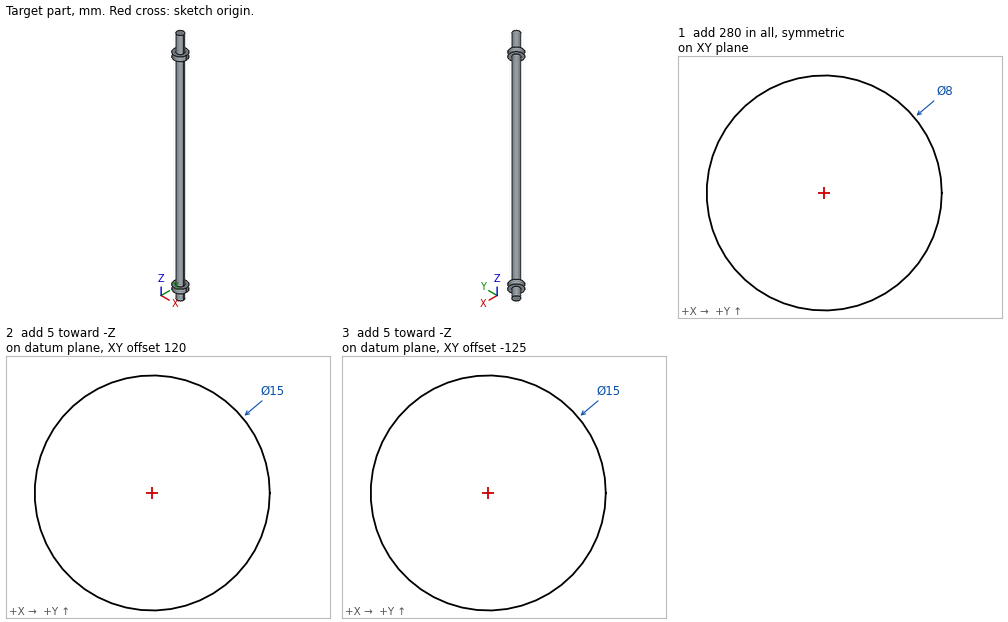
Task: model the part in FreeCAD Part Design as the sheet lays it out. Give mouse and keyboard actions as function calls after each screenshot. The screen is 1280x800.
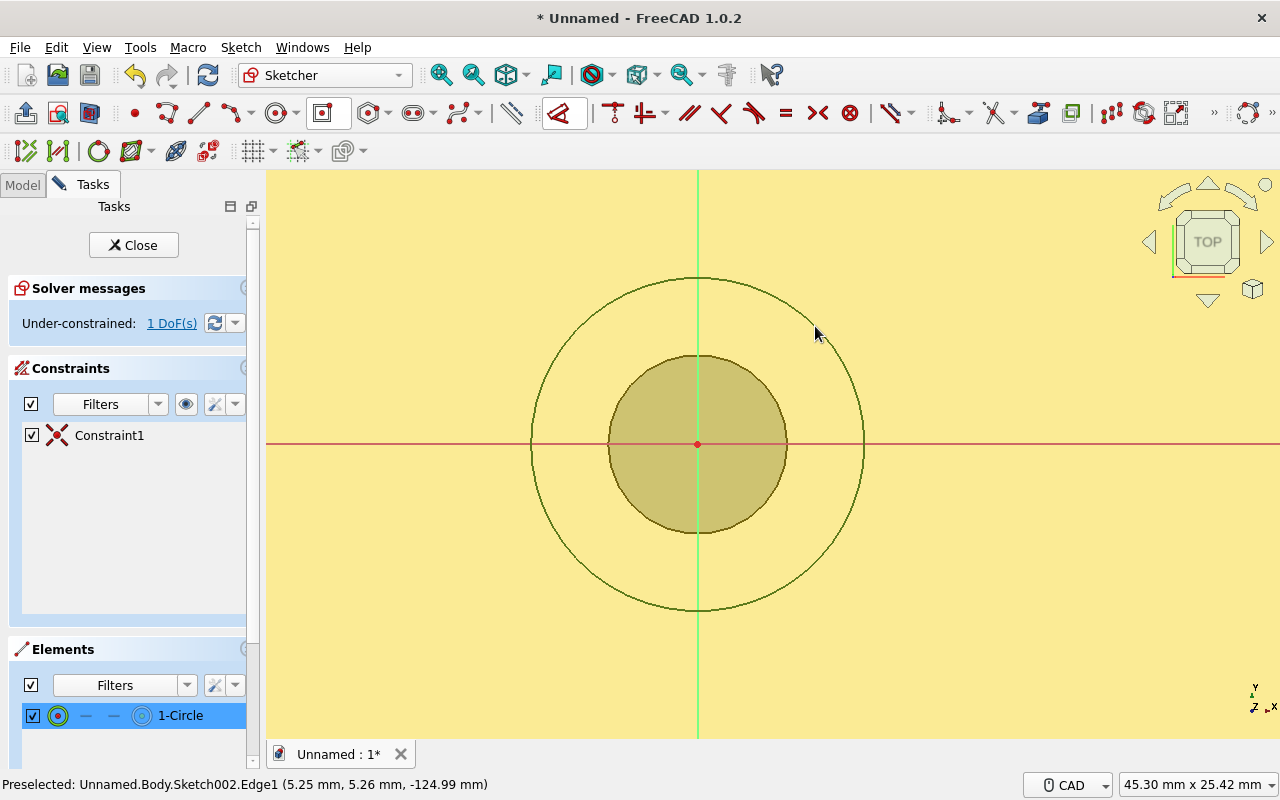
key(k)
key(o)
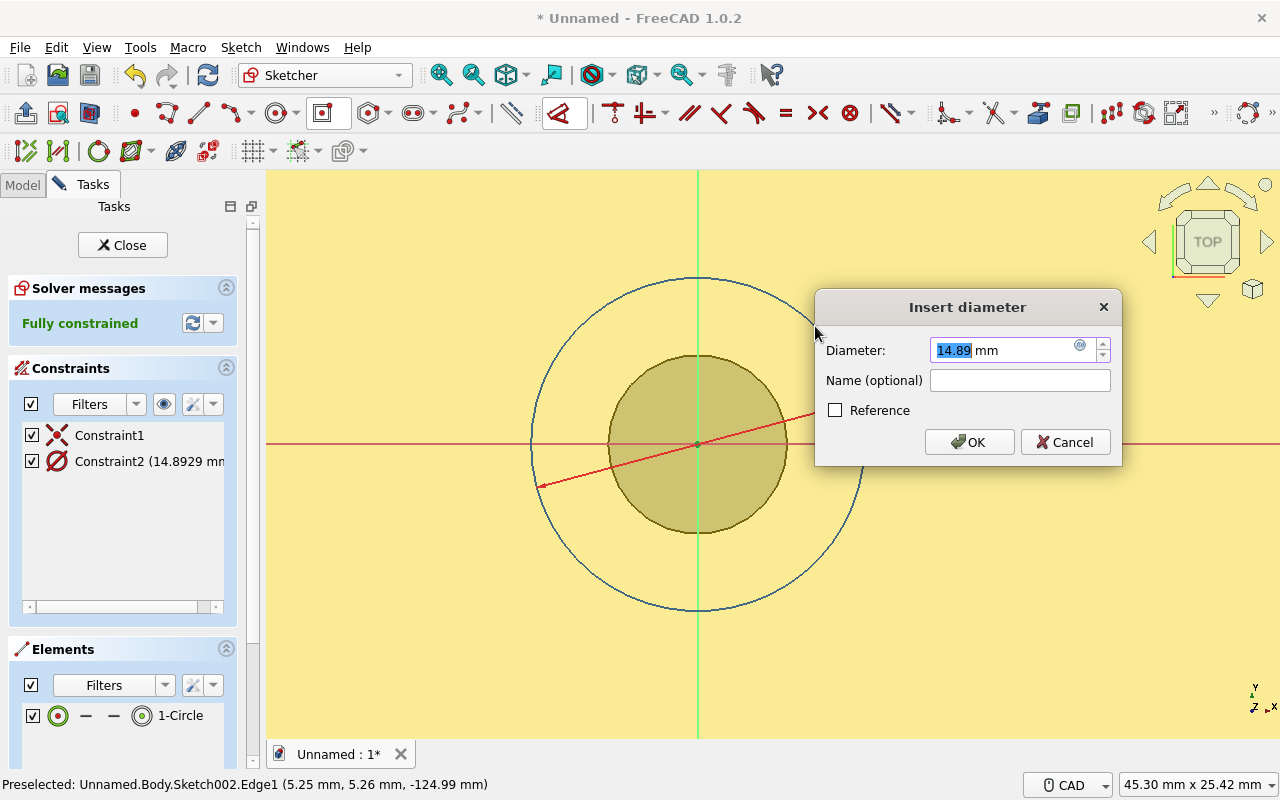
text(15)
key(Return)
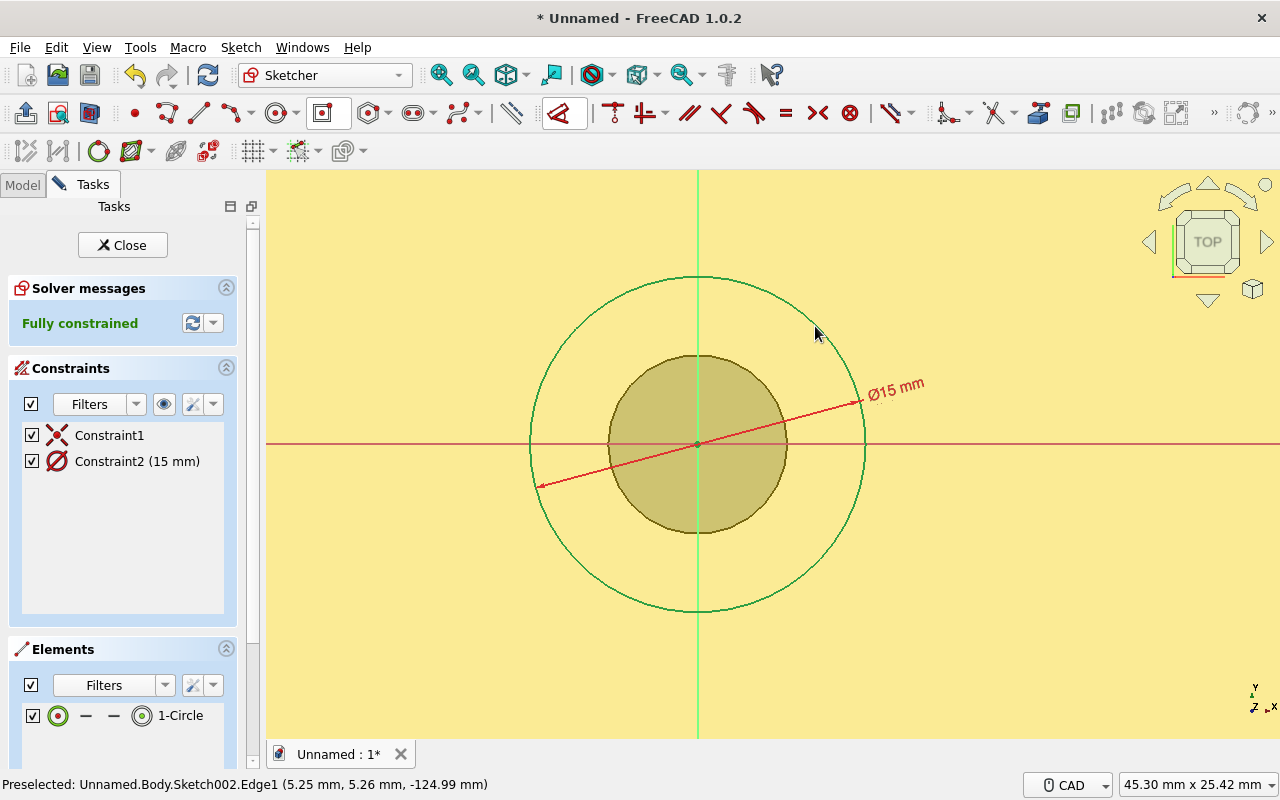
click(123, 245)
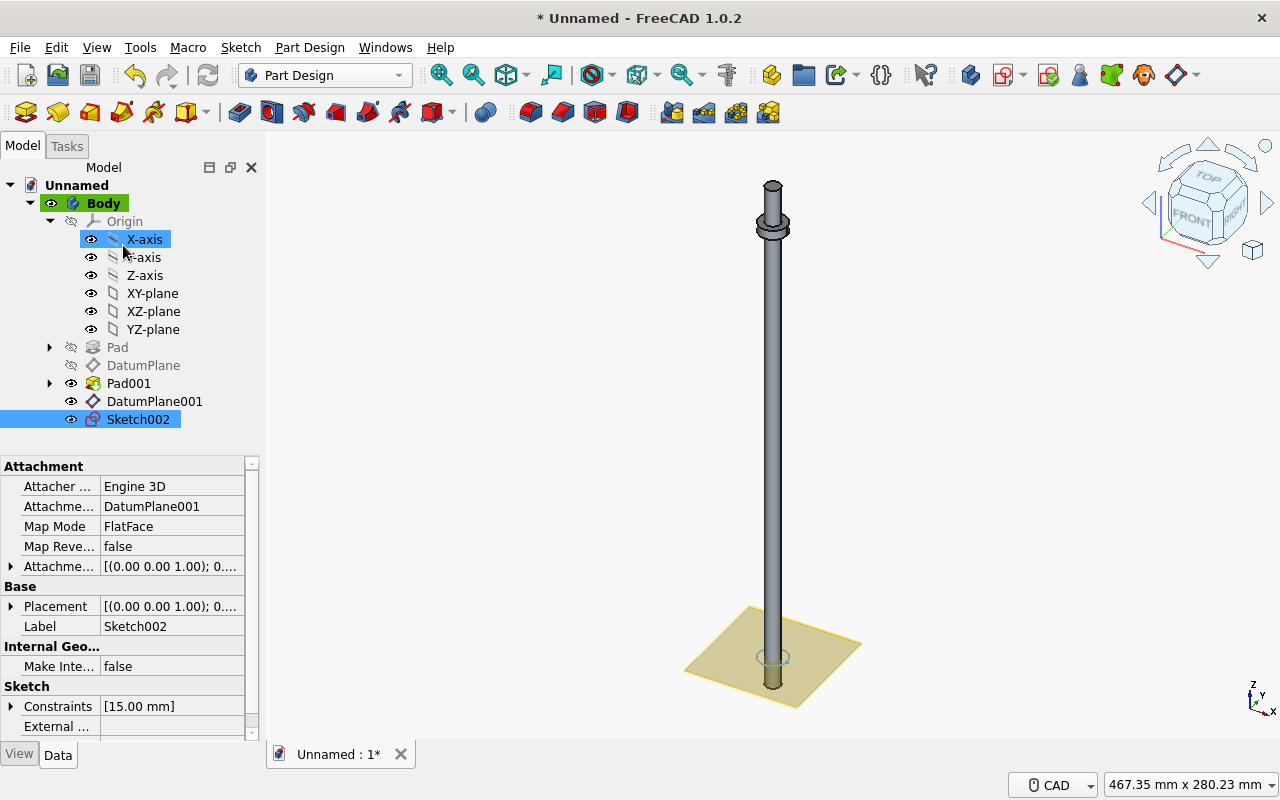
click(26, 112)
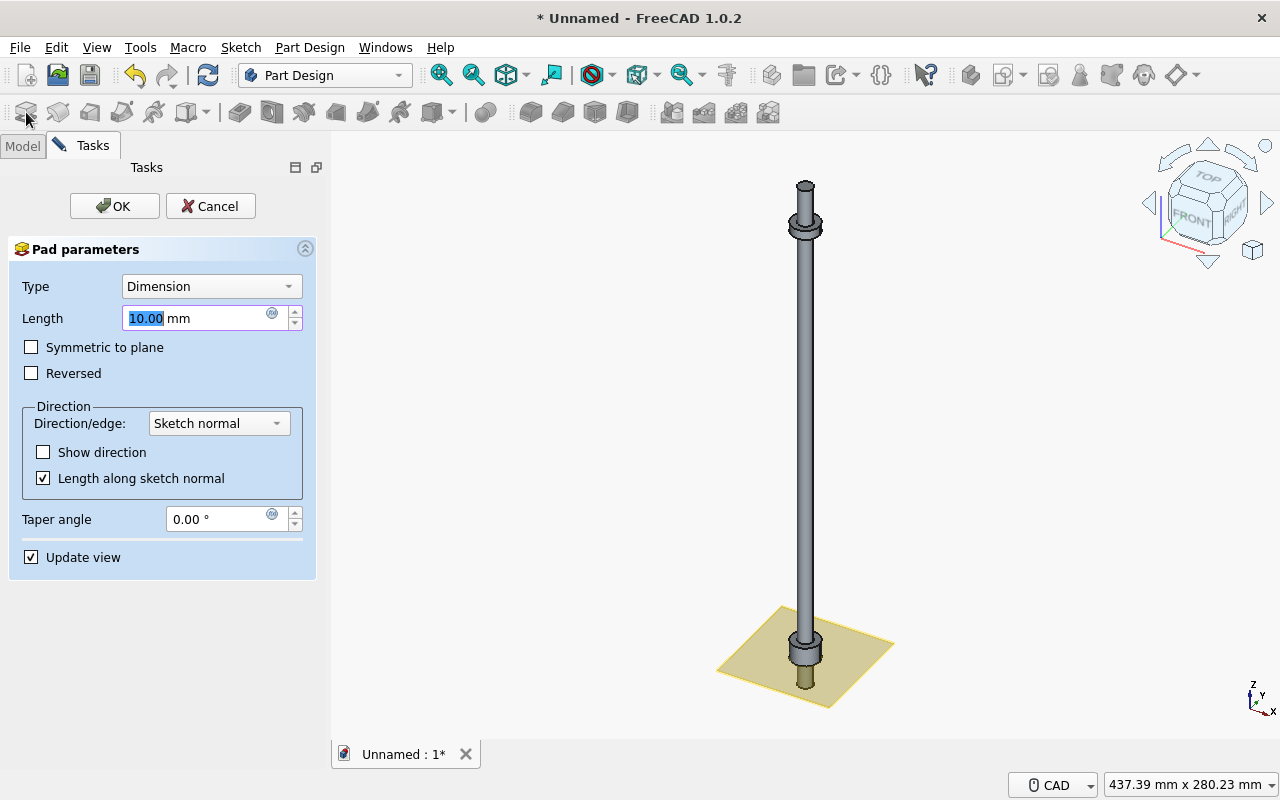
text(5)
key(Tab)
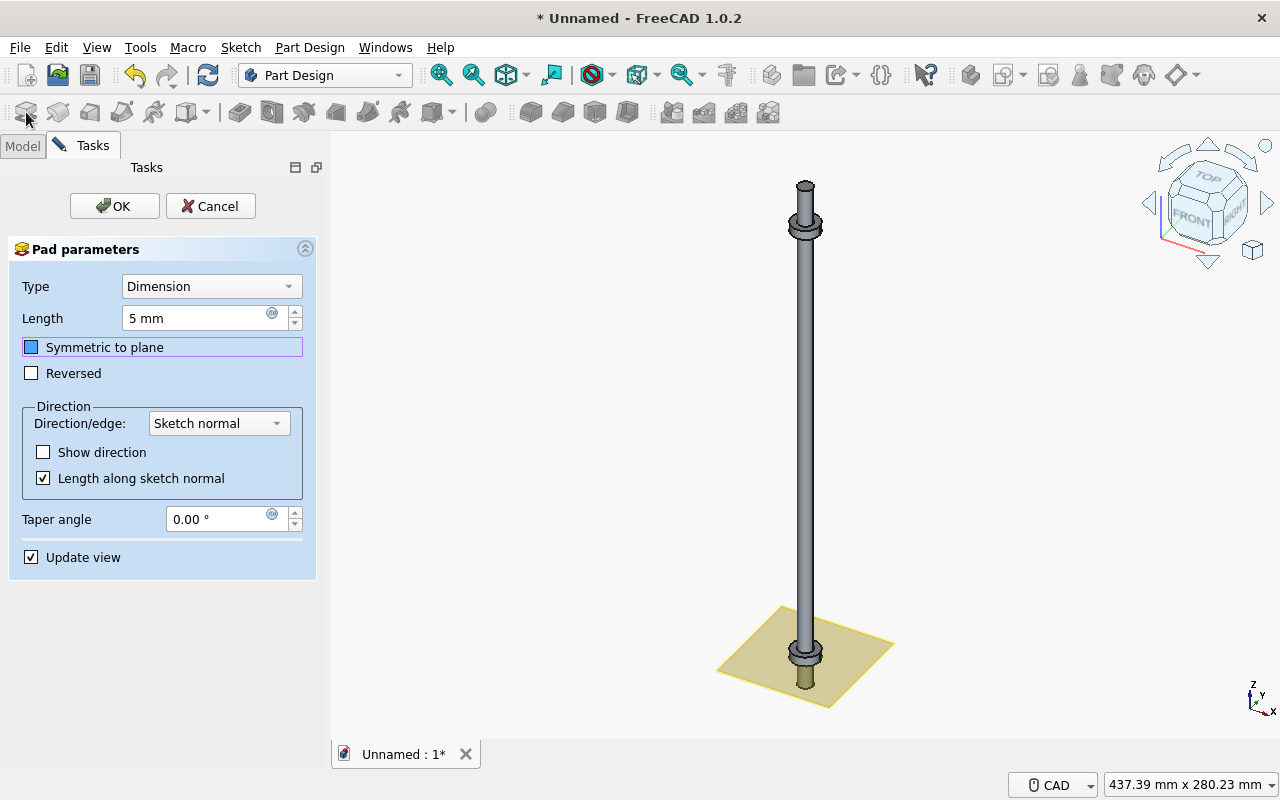
click(30, 373)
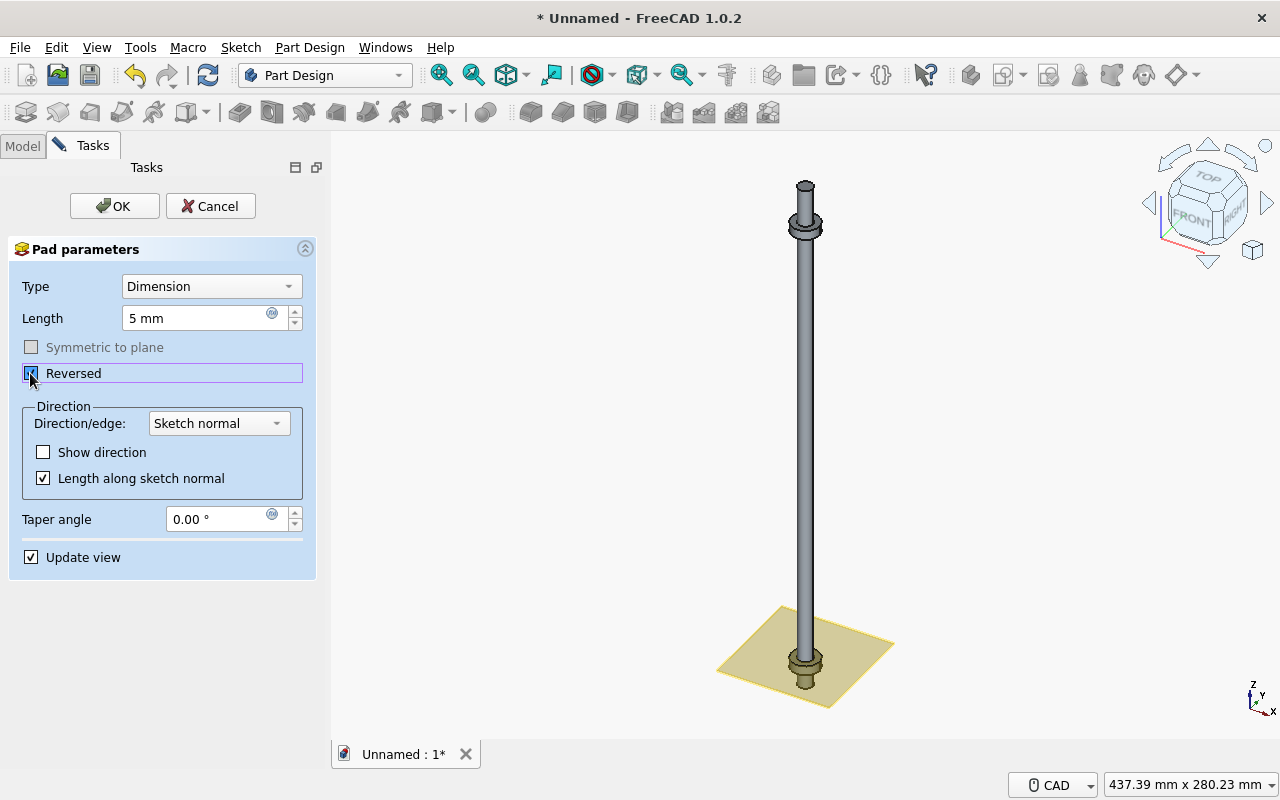
click(115, 206)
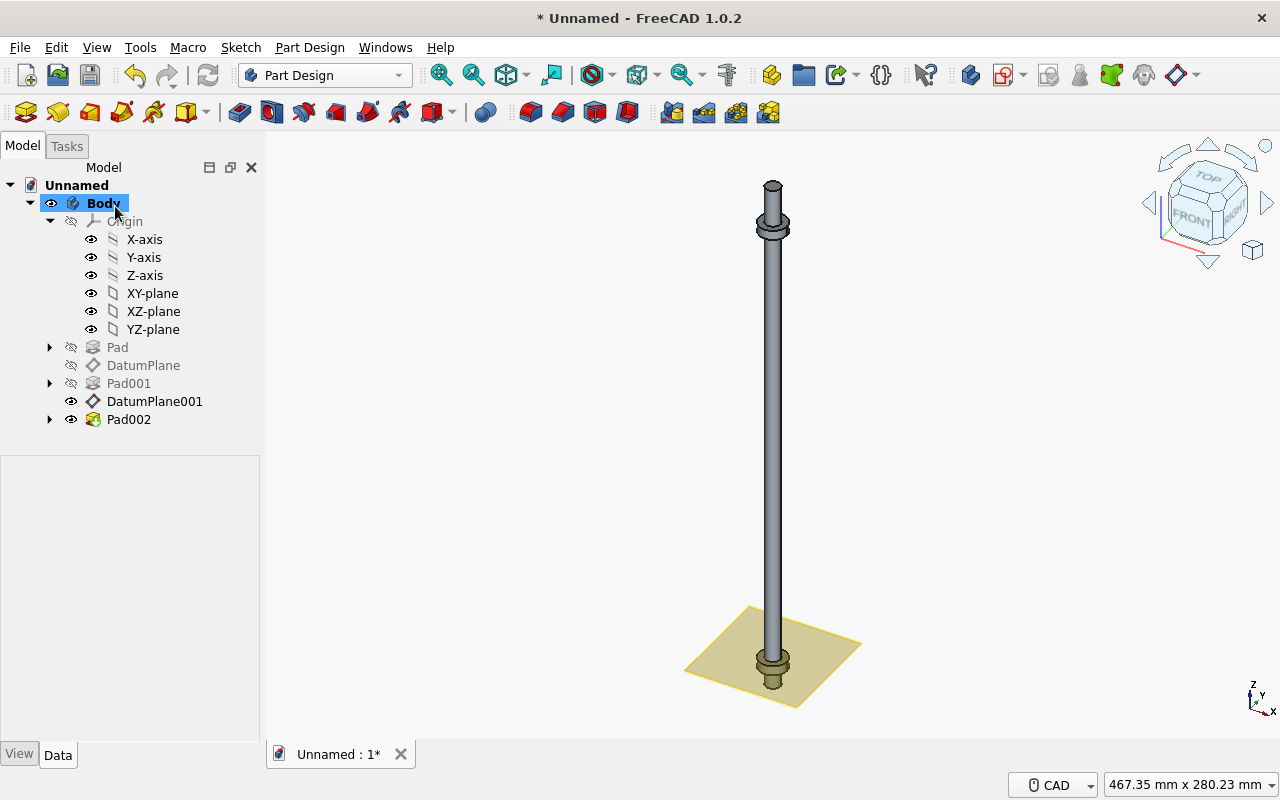
click(116, 401)
key(space)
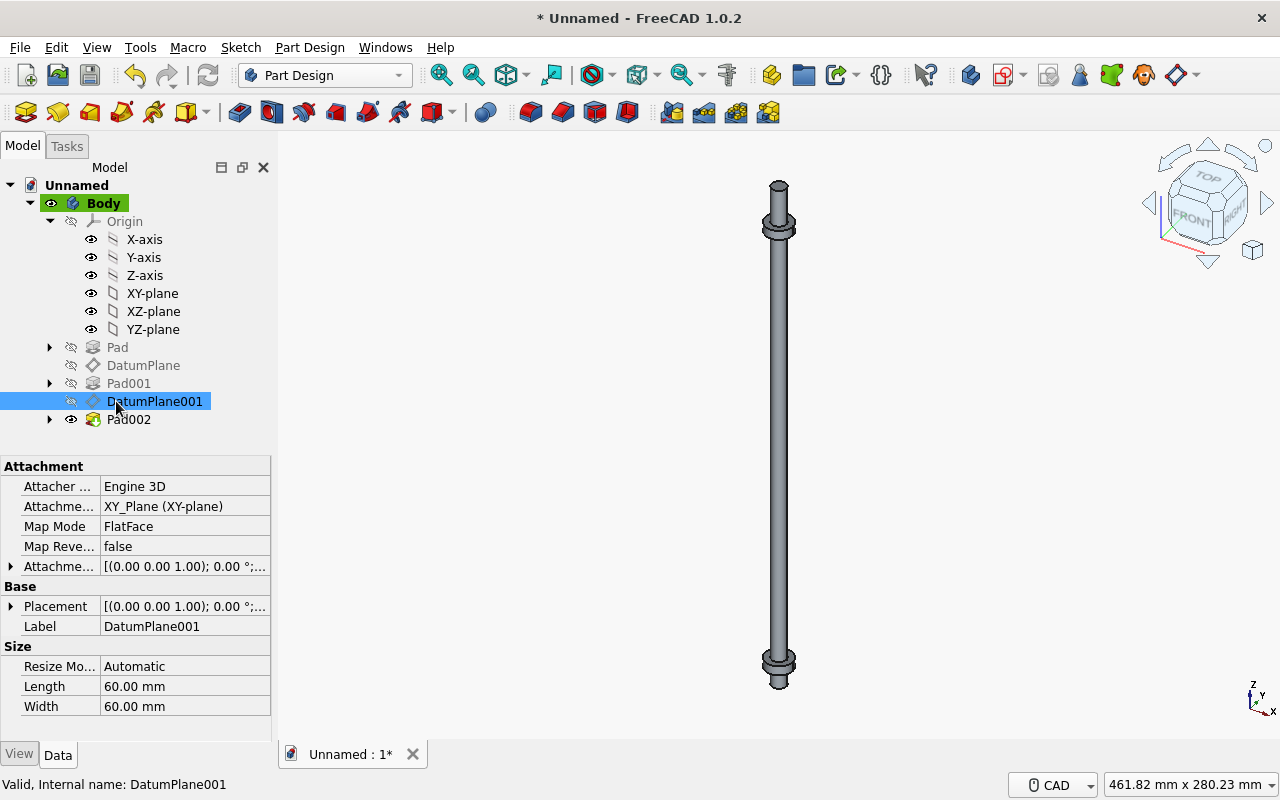
key(0)